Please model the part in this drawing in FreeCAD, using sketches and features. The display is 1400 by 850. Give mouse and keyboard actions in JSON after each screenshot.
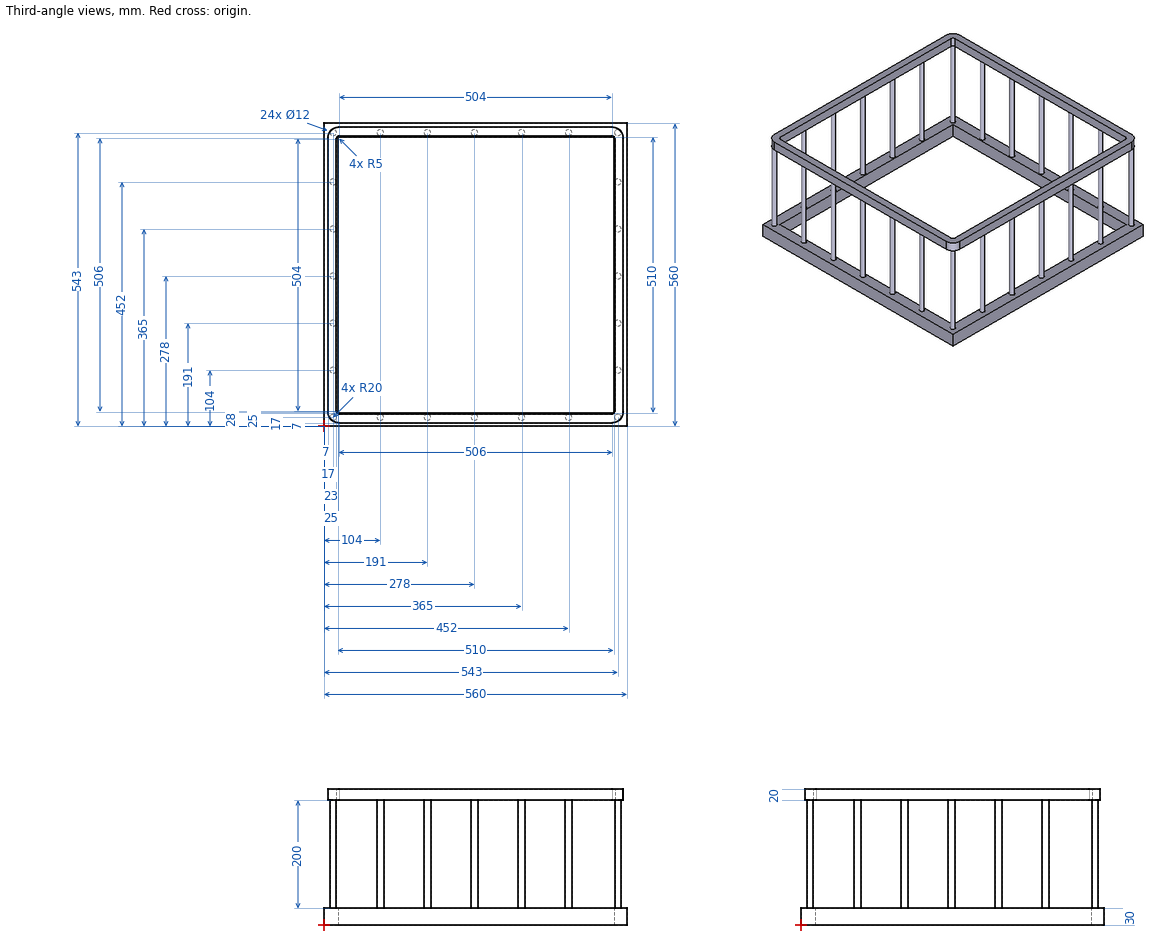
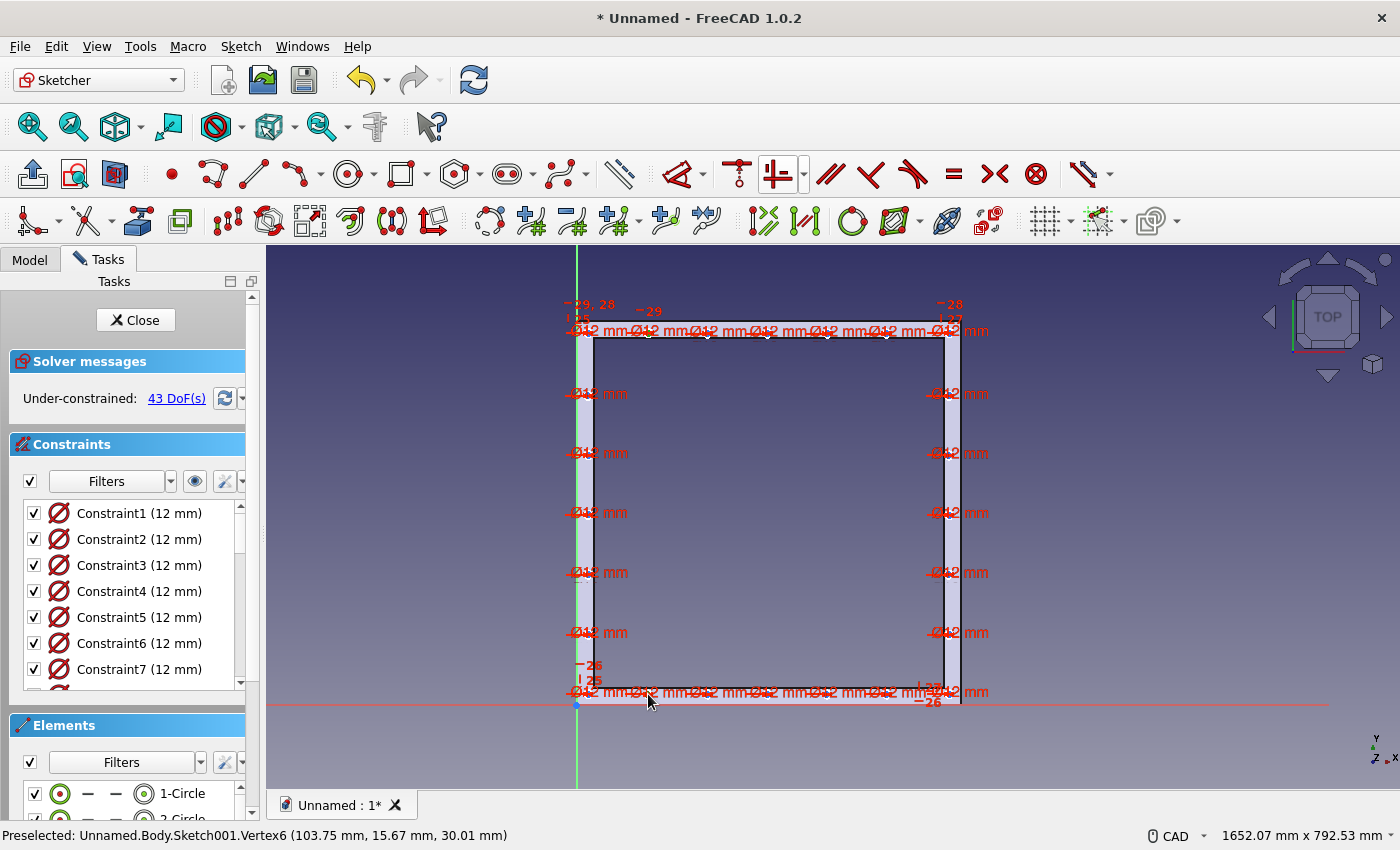
{"action": "key", "text": "v"}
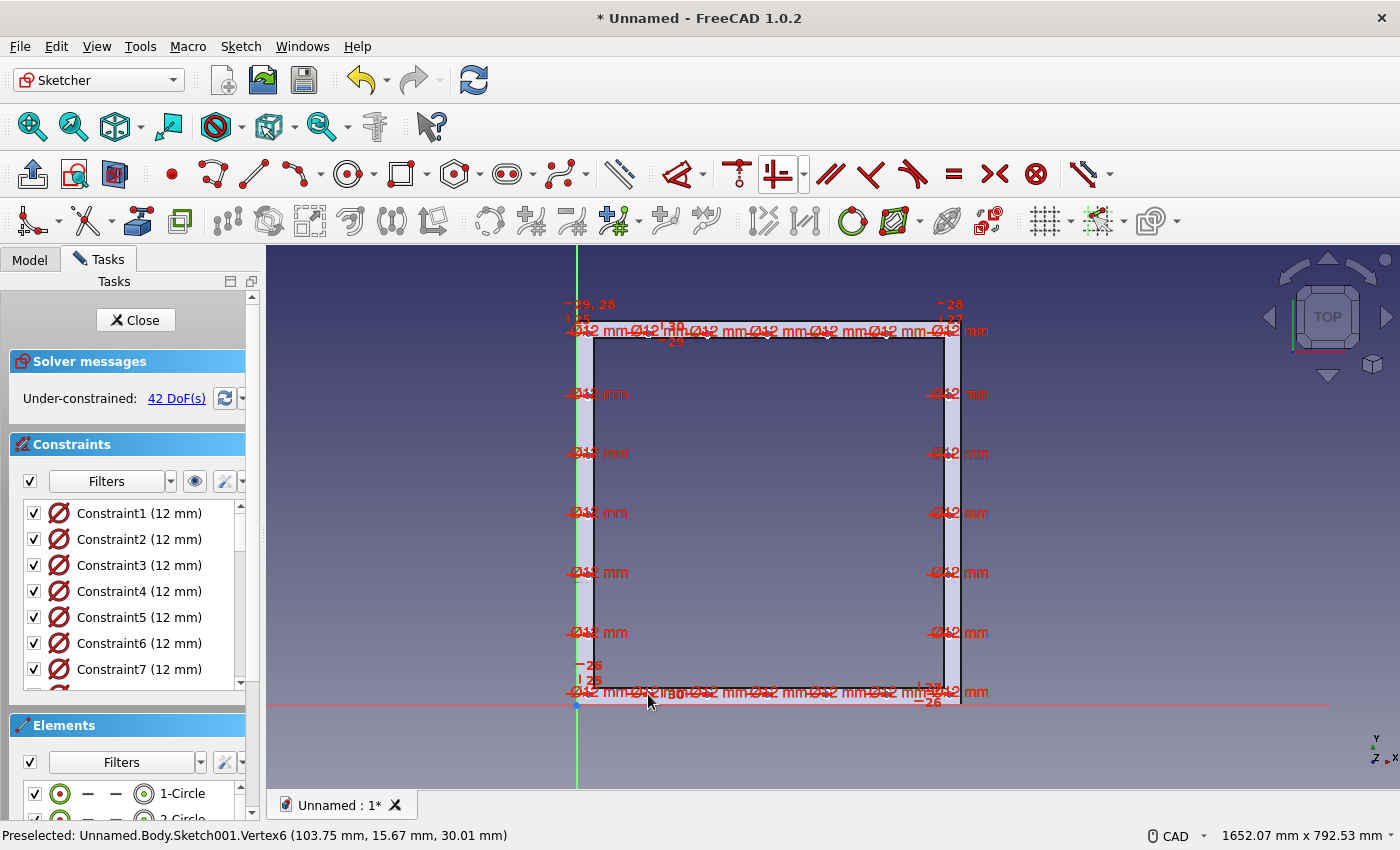
{"action": "left_click", "coordinate": [588, 694]}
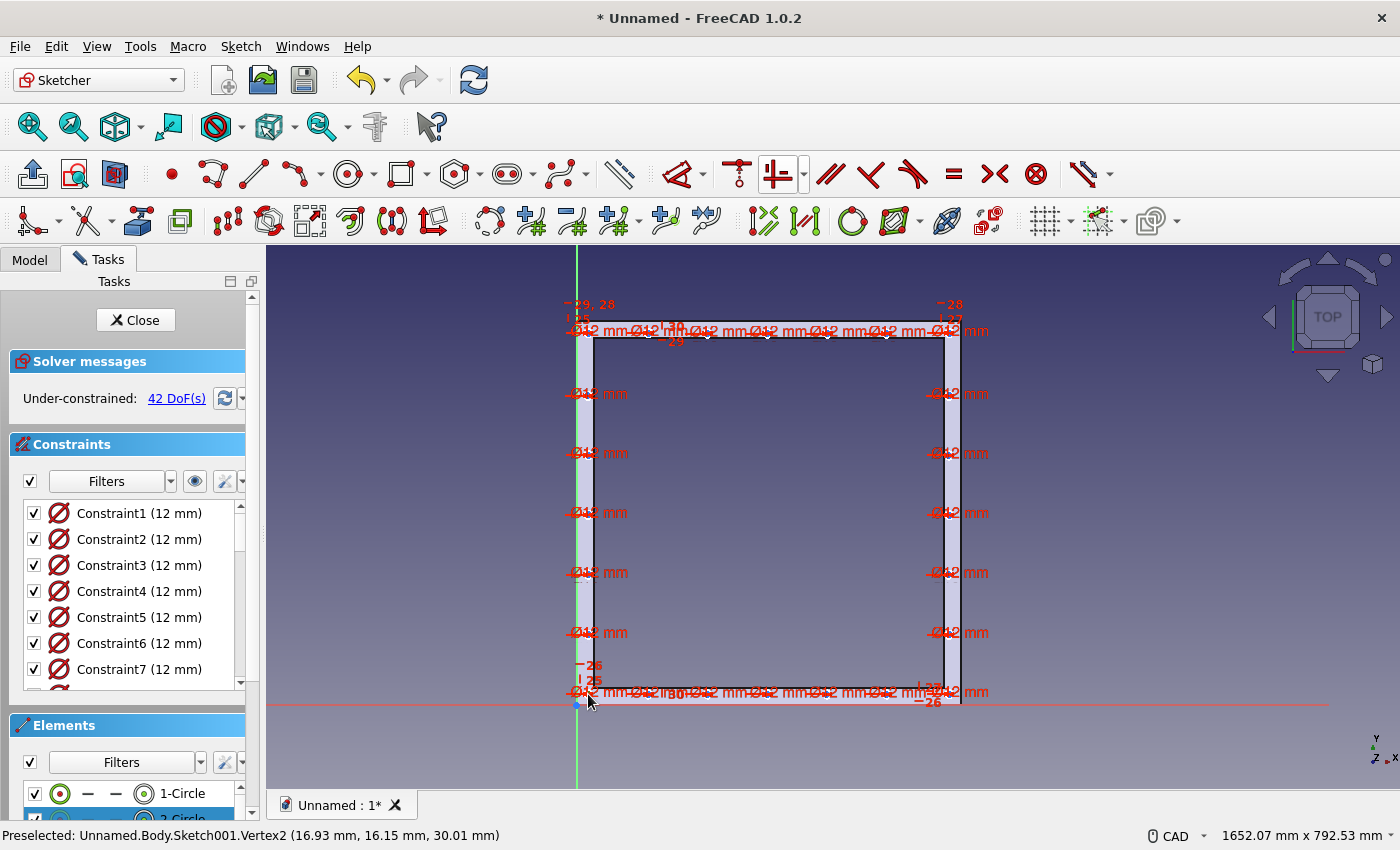
{"action": "left_click", "coordinate": [648, 694]}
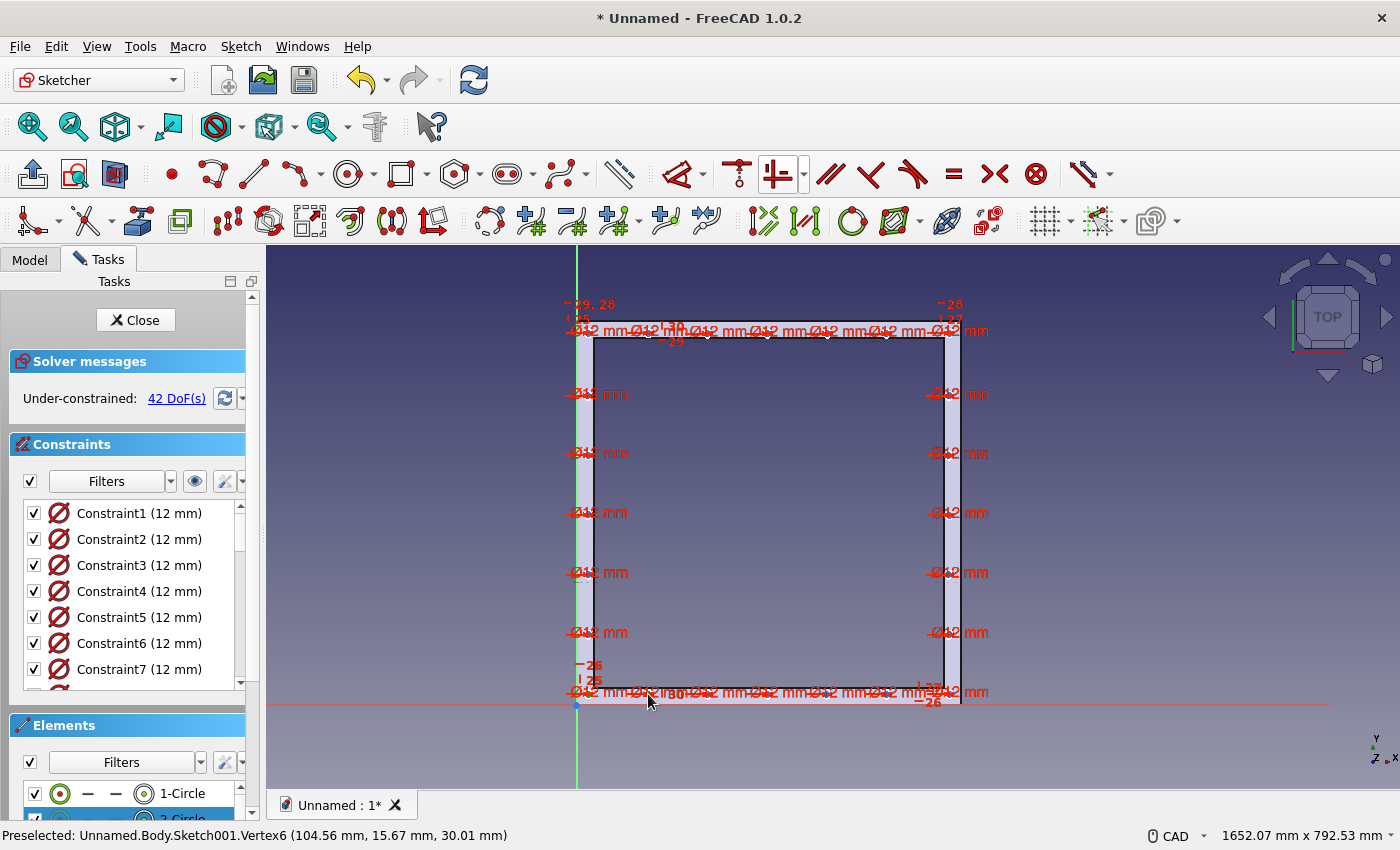
{"action": "key", "text": "h"}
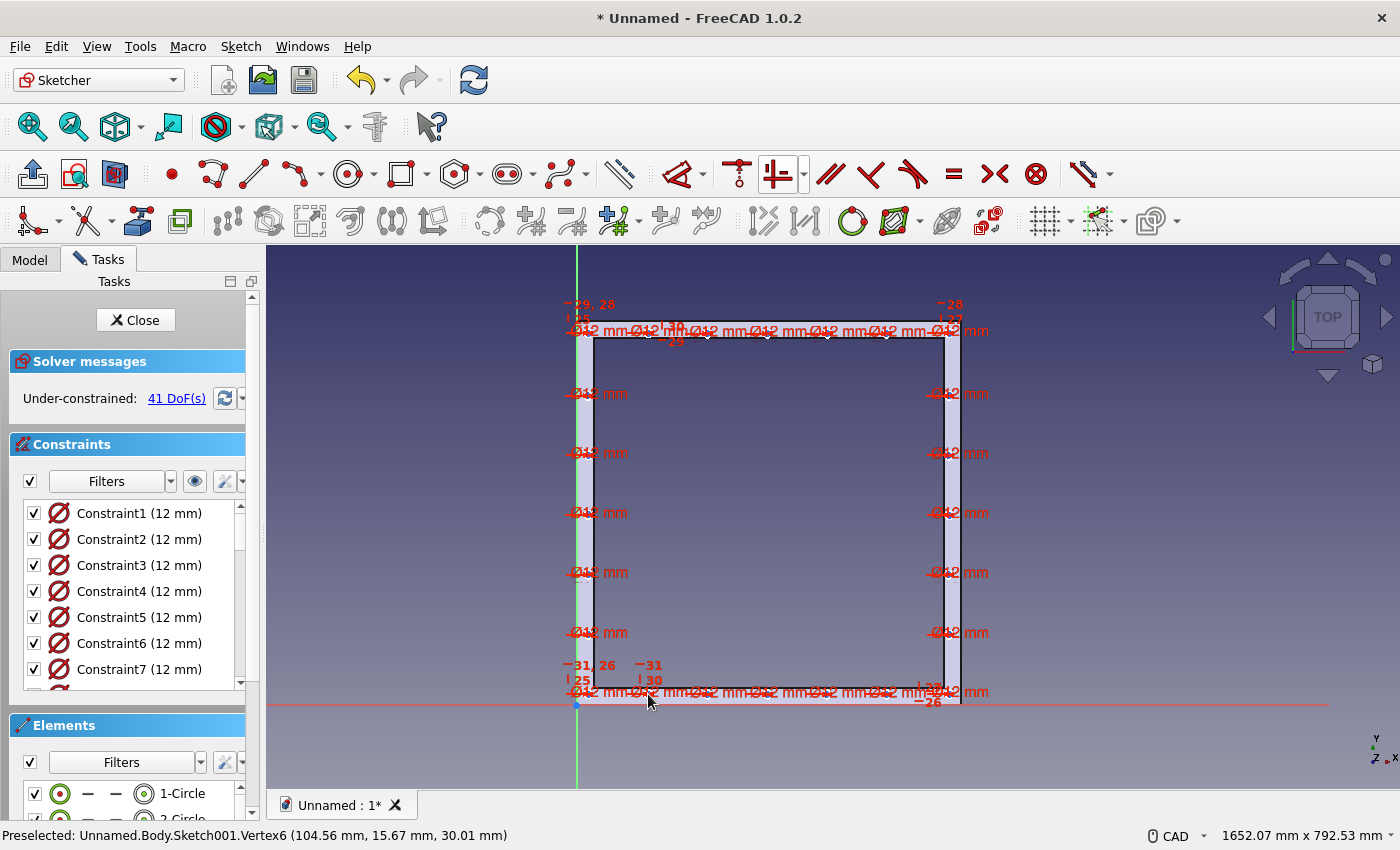
{"action": "left_click", "coordinate": [648, 333]}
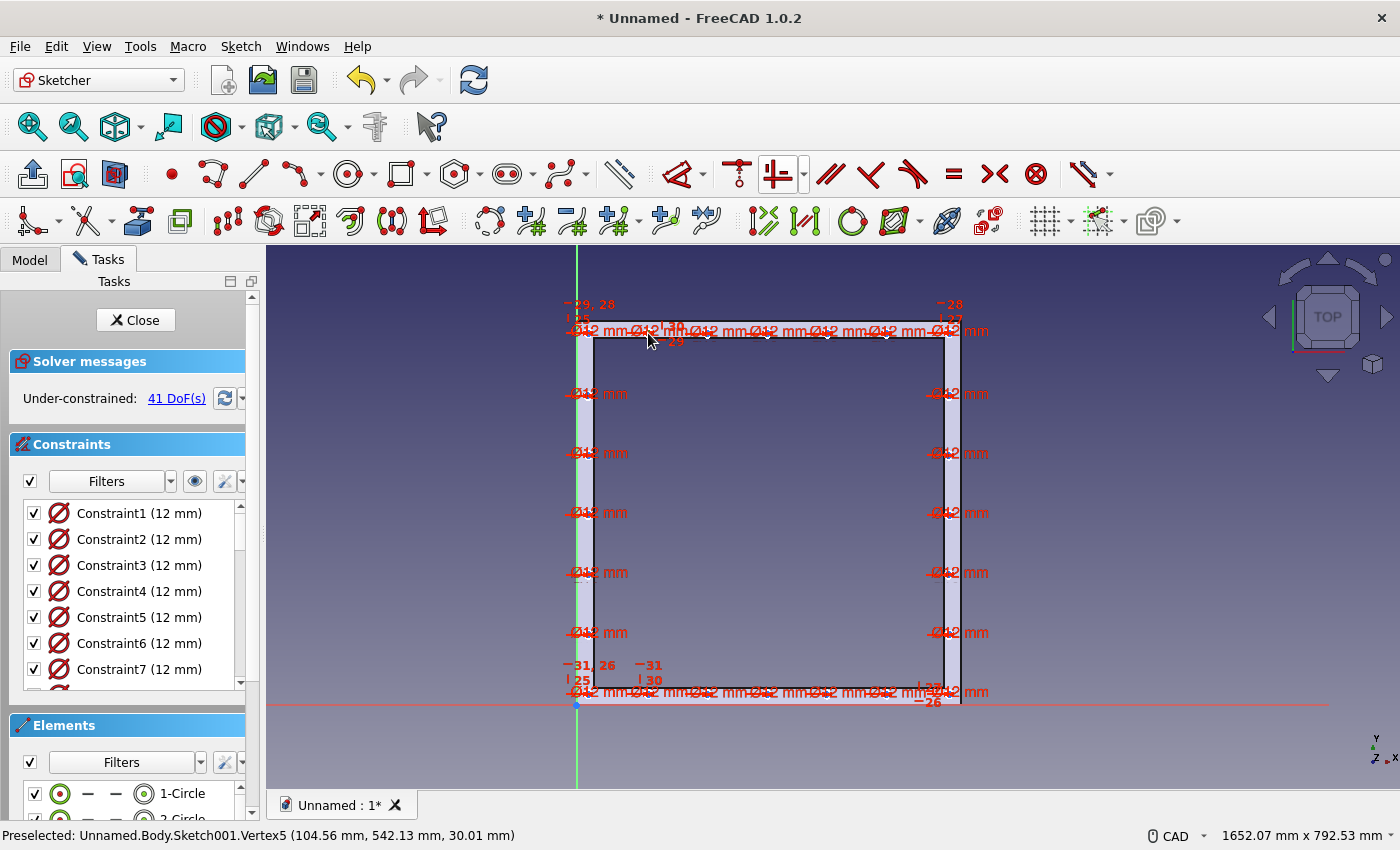
{"action": "left_click", "coordinate": [707, 334]}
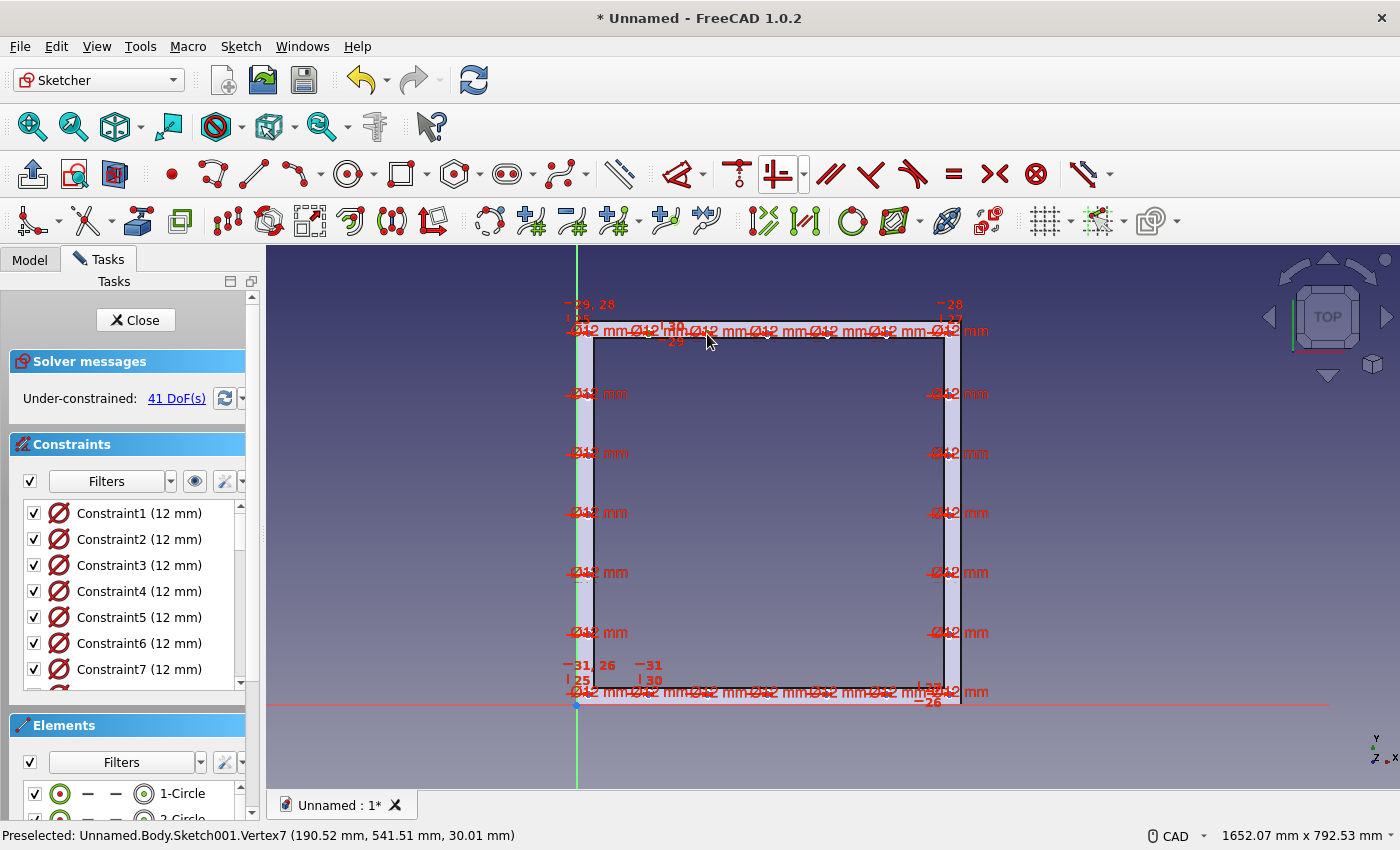
{"action": "key", "text": "h"}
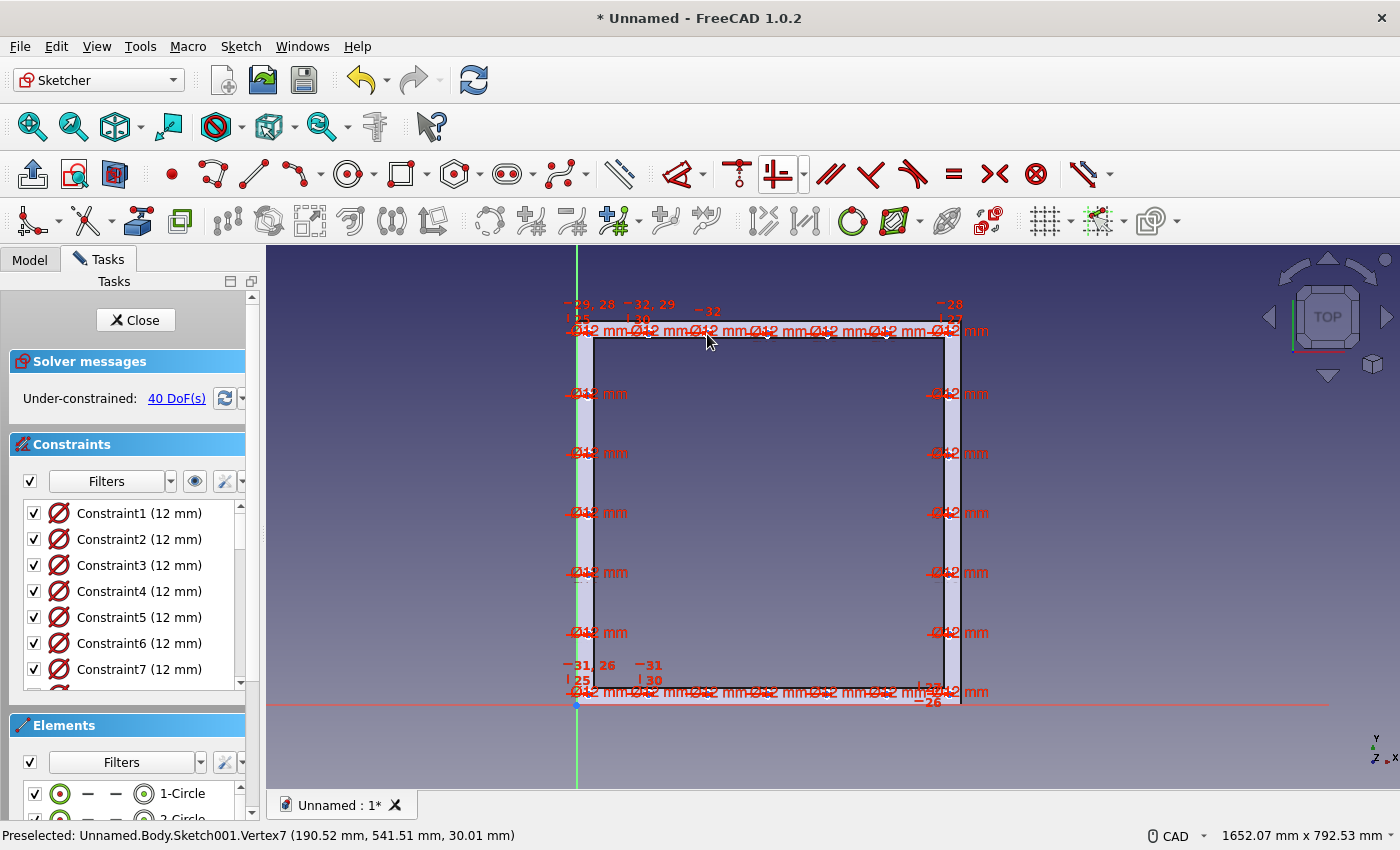
{"action": "left_click", "coordinate": [707, 333]}